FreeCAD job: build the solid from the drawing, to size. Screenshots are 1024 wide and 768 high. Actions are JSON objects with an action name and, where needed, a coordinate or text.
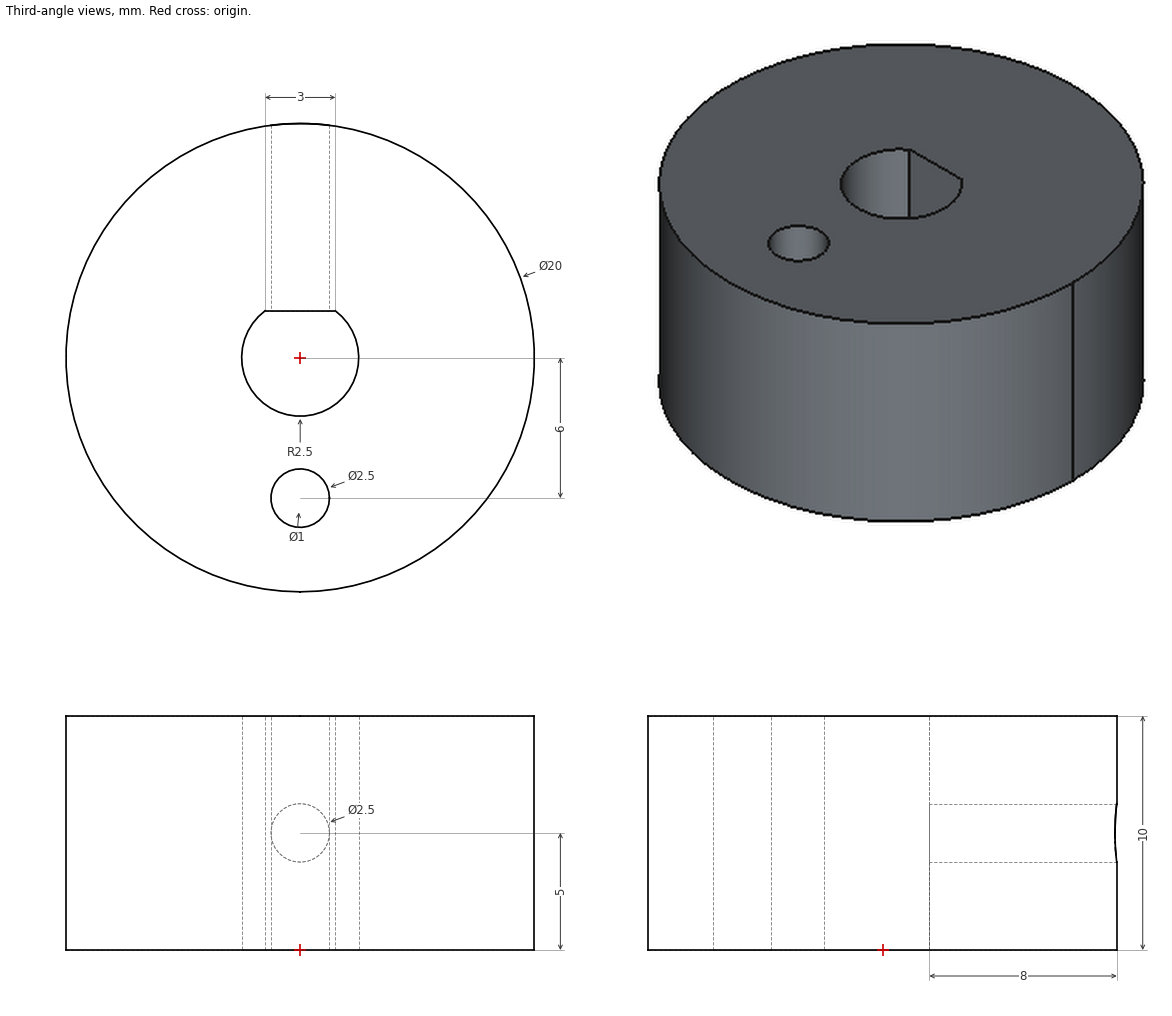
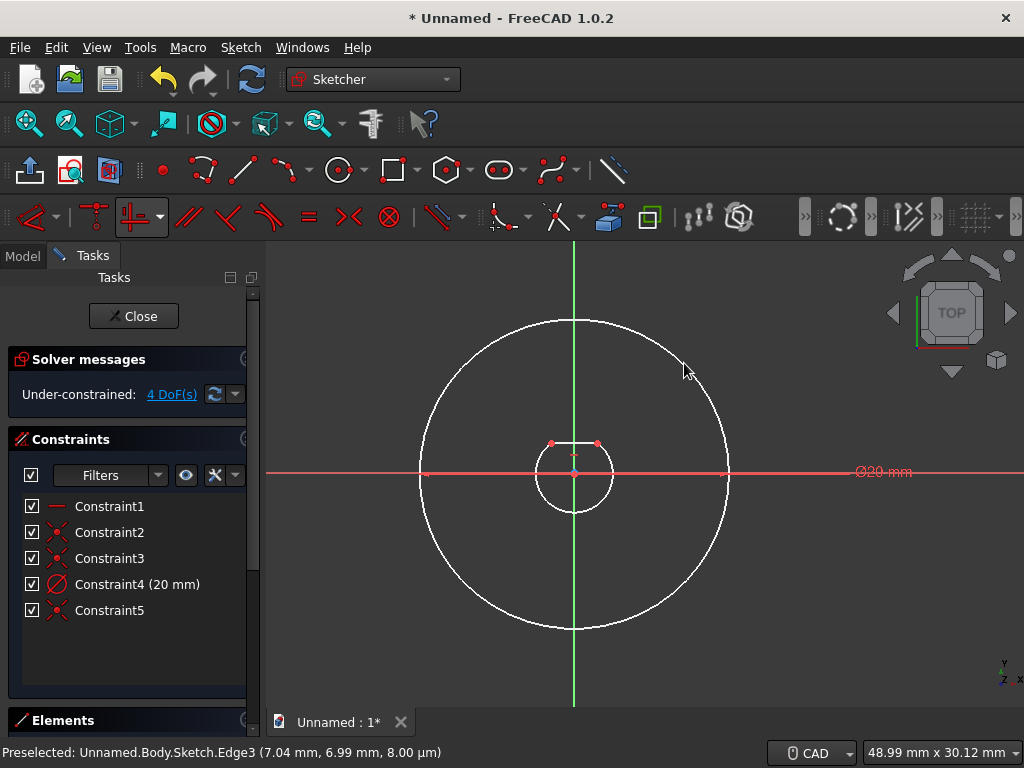
{"action": "left_click_drag", "start_coordinate": [564, 463], "coordinate": [584, 484]}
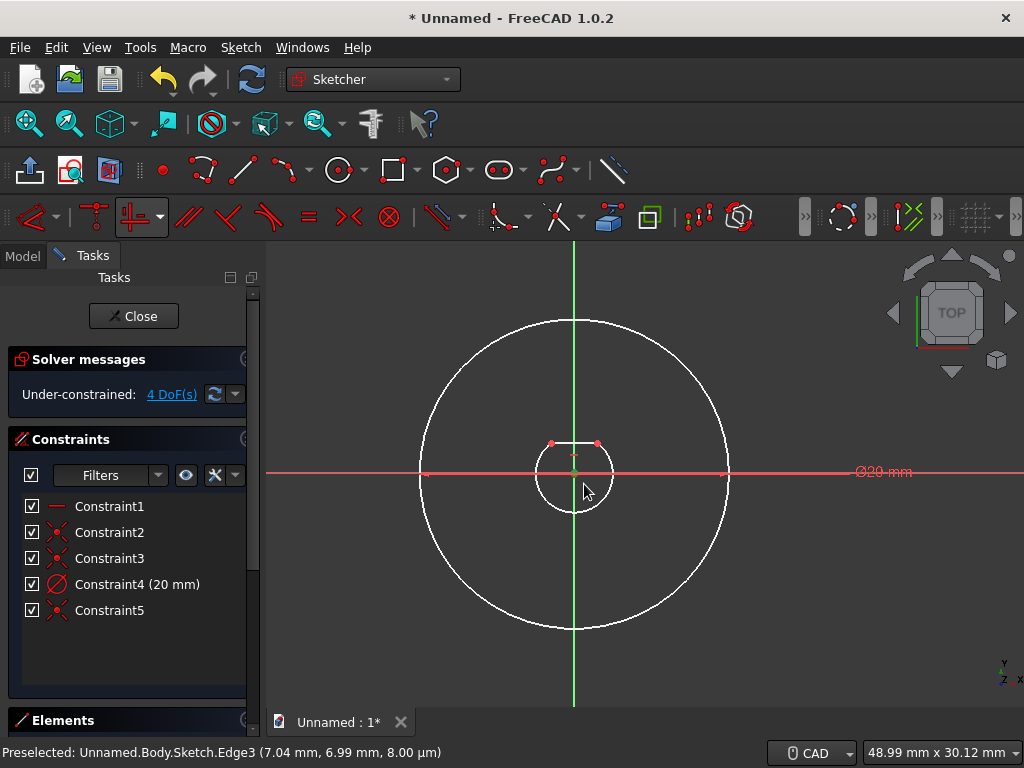
{"action": "left_click", "coordinate": [94, 218]}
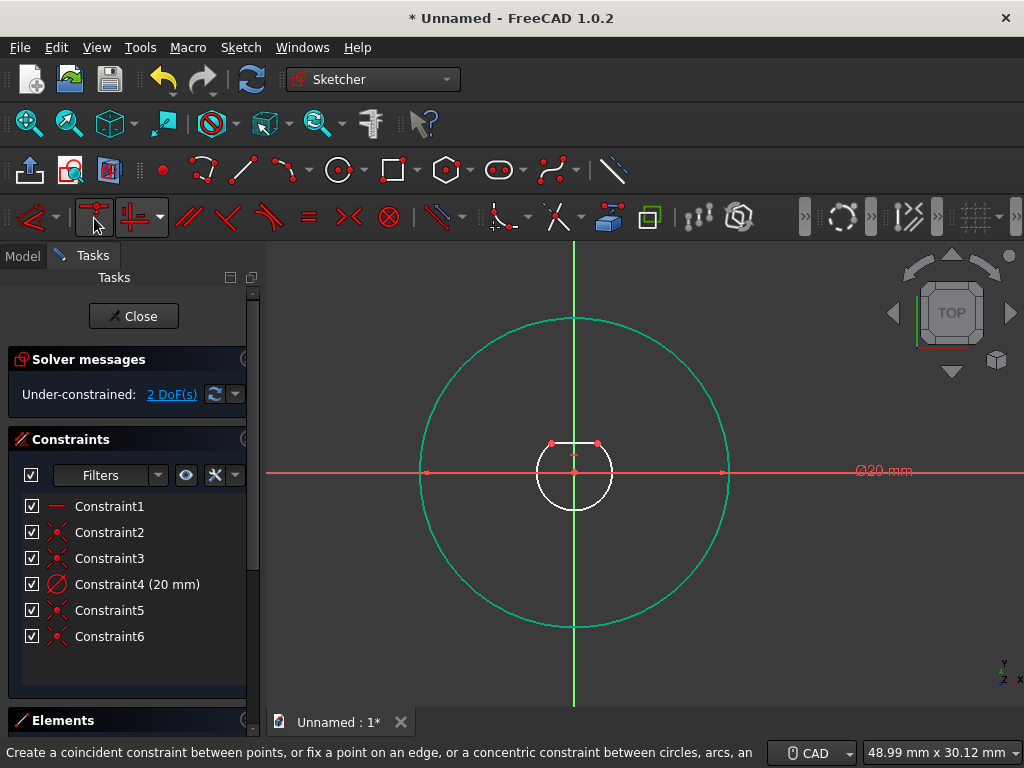
{"action": "left_click", "coordinate": [32, 218]}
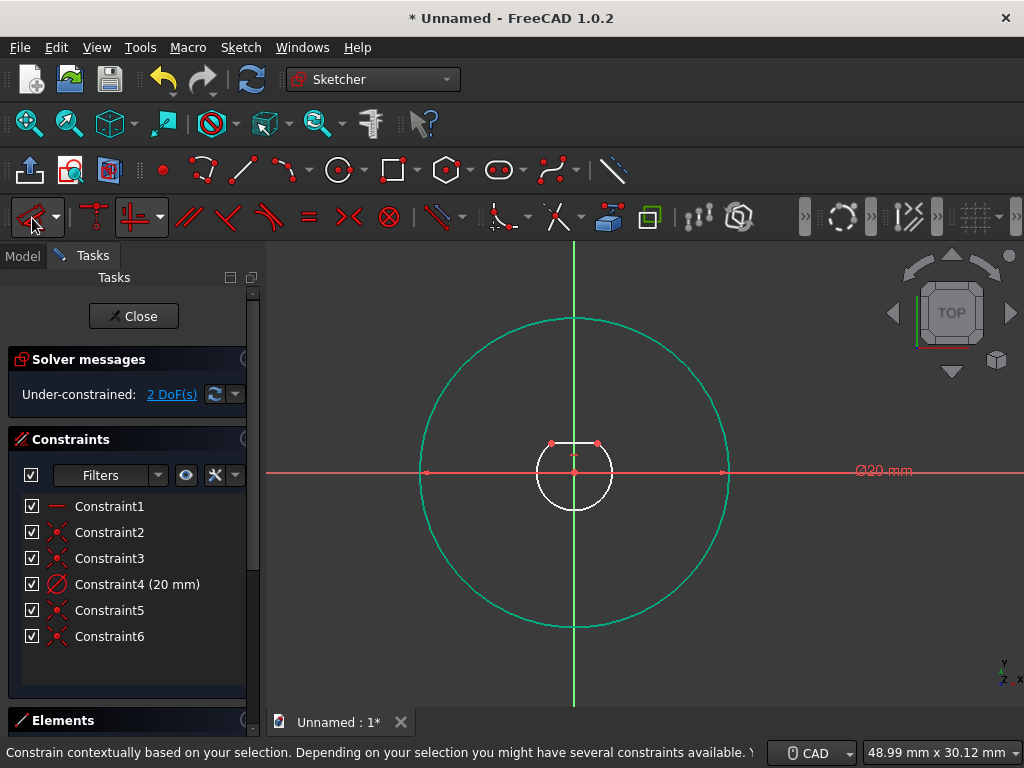
{"action": "left_click", "coordinate": [543, 493]}
{"action": "left_click", "coordinate": [516, 510]}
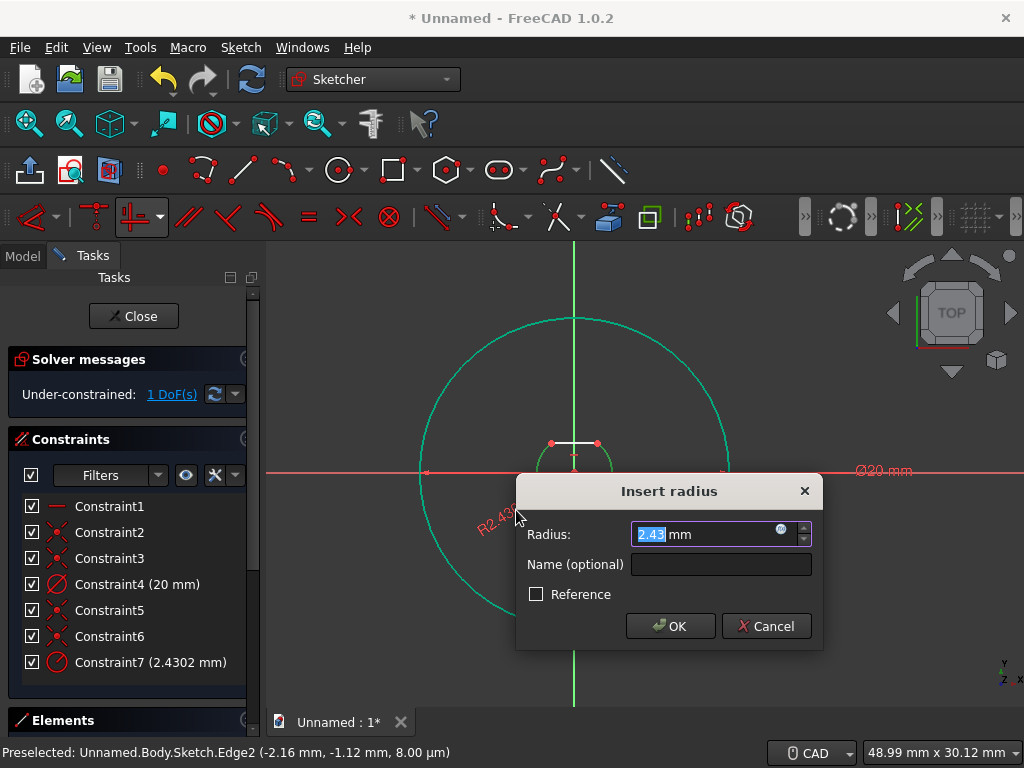
{"action": "type", "text": "2.5"}
{"action": "key", "text": "Return"}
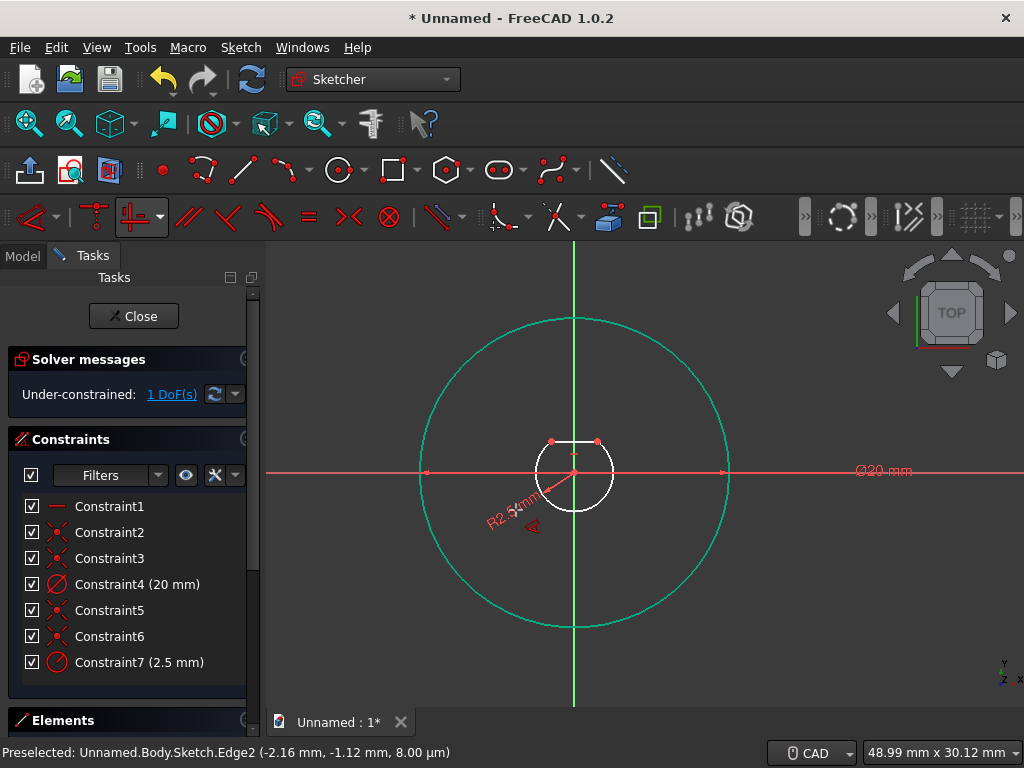
{"action": "scroll", "coordinate": [584, 442], "scroll_direction": "up", "scroll_amount": 3}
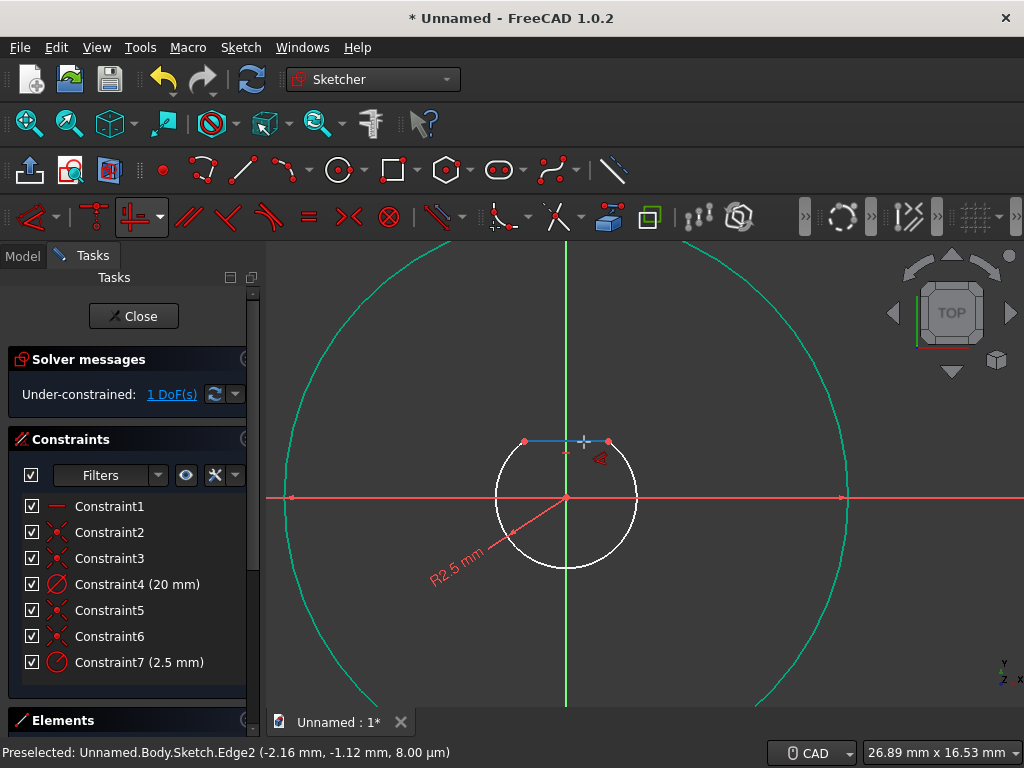
{"action": "left_click", "coordinate": [583, 441]}
{"action": "left_click", "coordinate": [547, 407]}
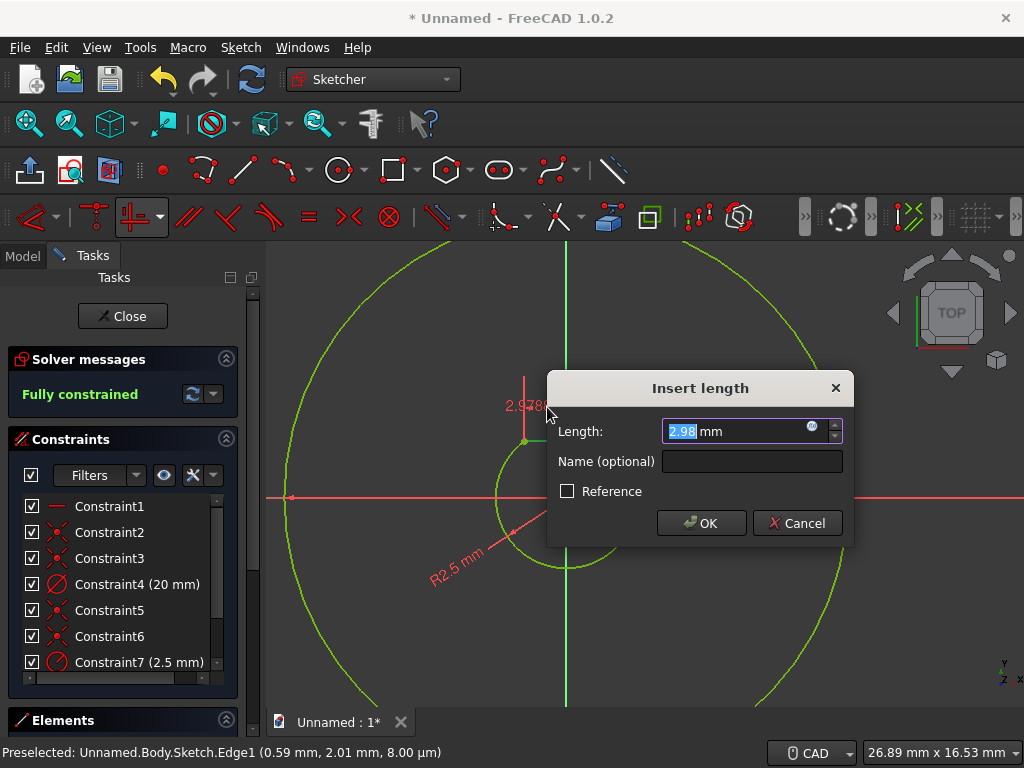
{"action": "type", "text": "3"}
{"action": "key", "text": "Return"}
{"action": "key", "text": "Escape"}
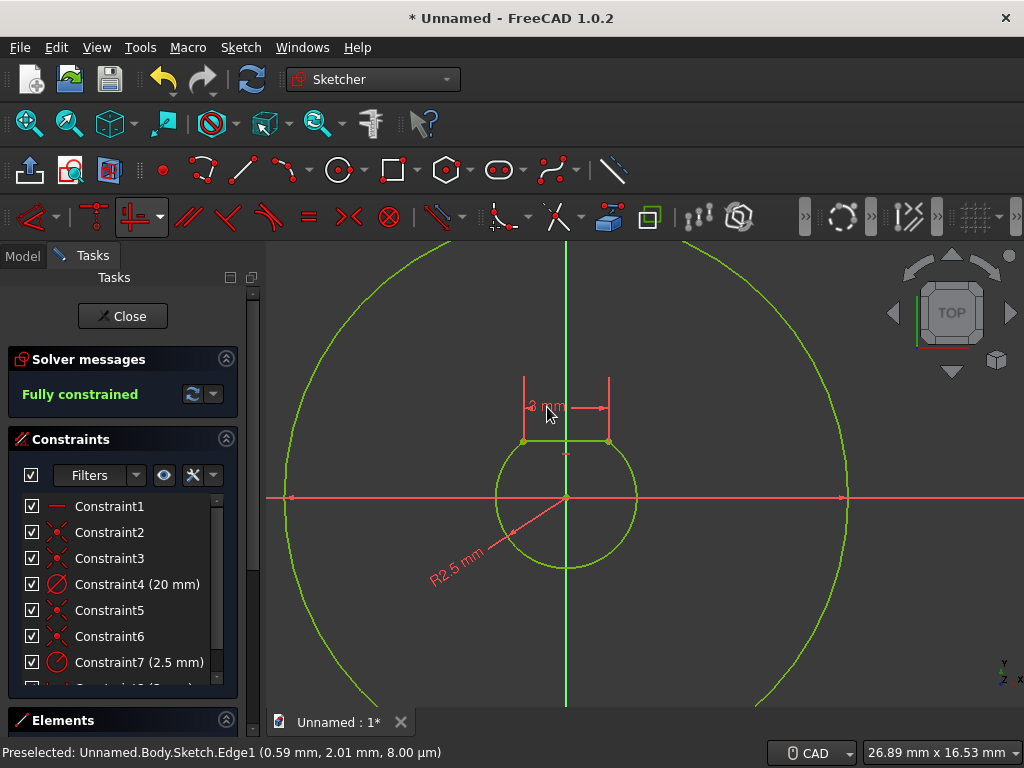
{"action": "left_click", "coordinate": [123, 316]}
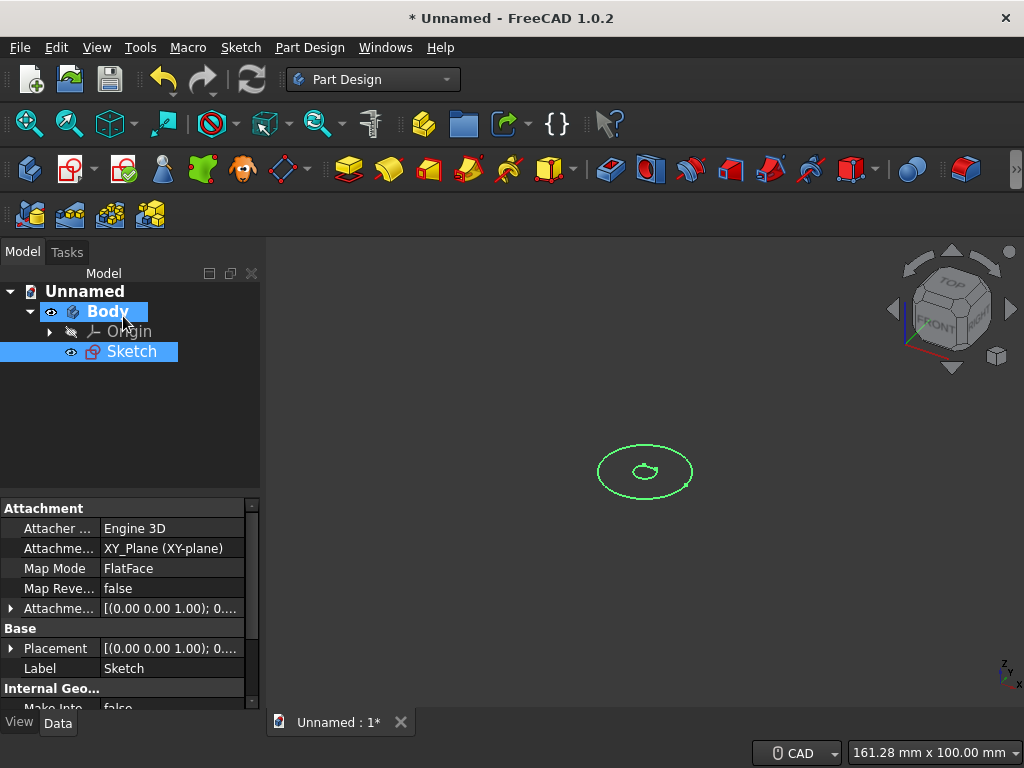
{"action": "left_click", "coordinate": [350, 170]}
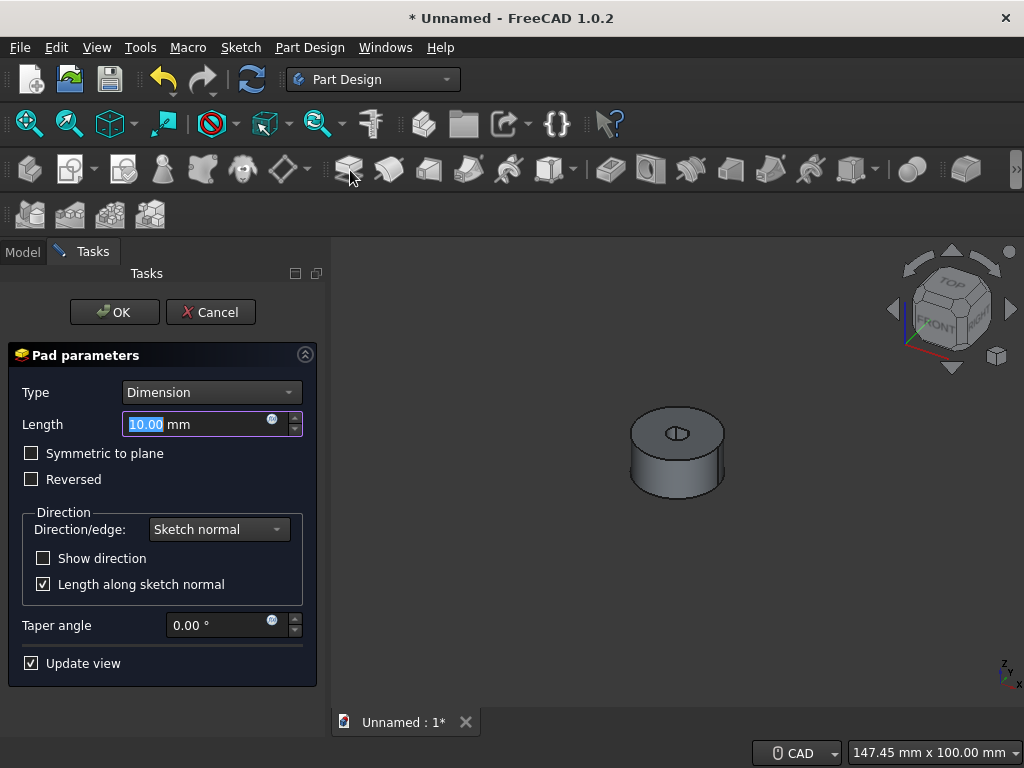
{"action": "type", "text": "10"}
{"action": "key", "text": "Tab"}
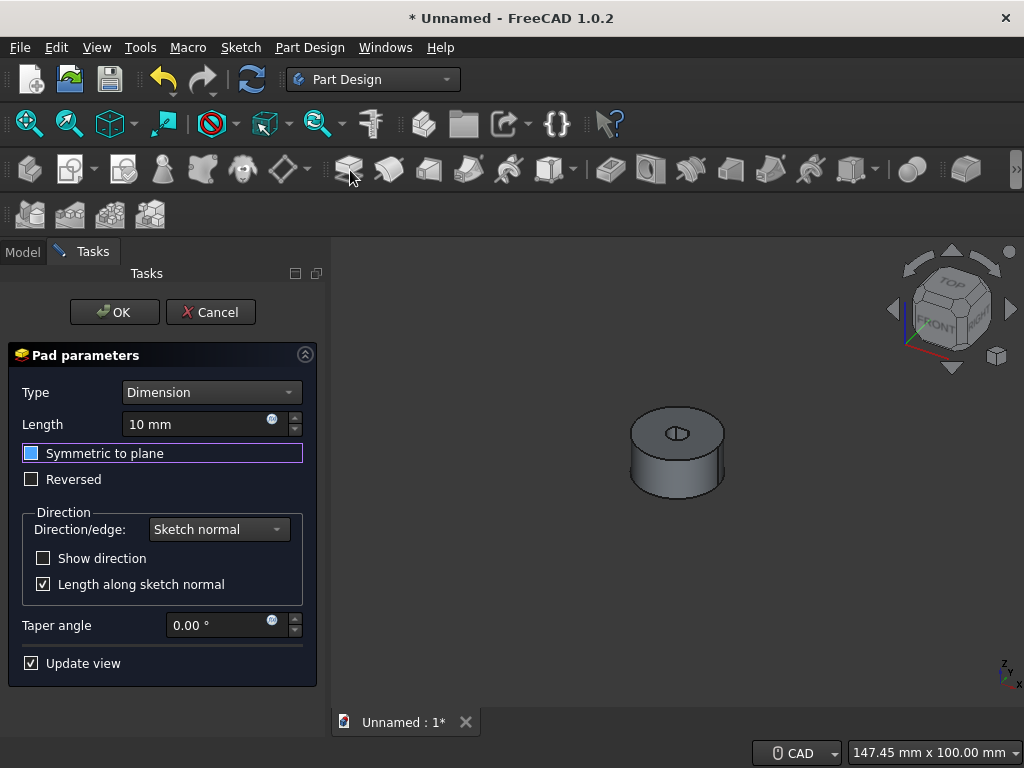
{"action": "left_click", "coordinate": [115, 312]}